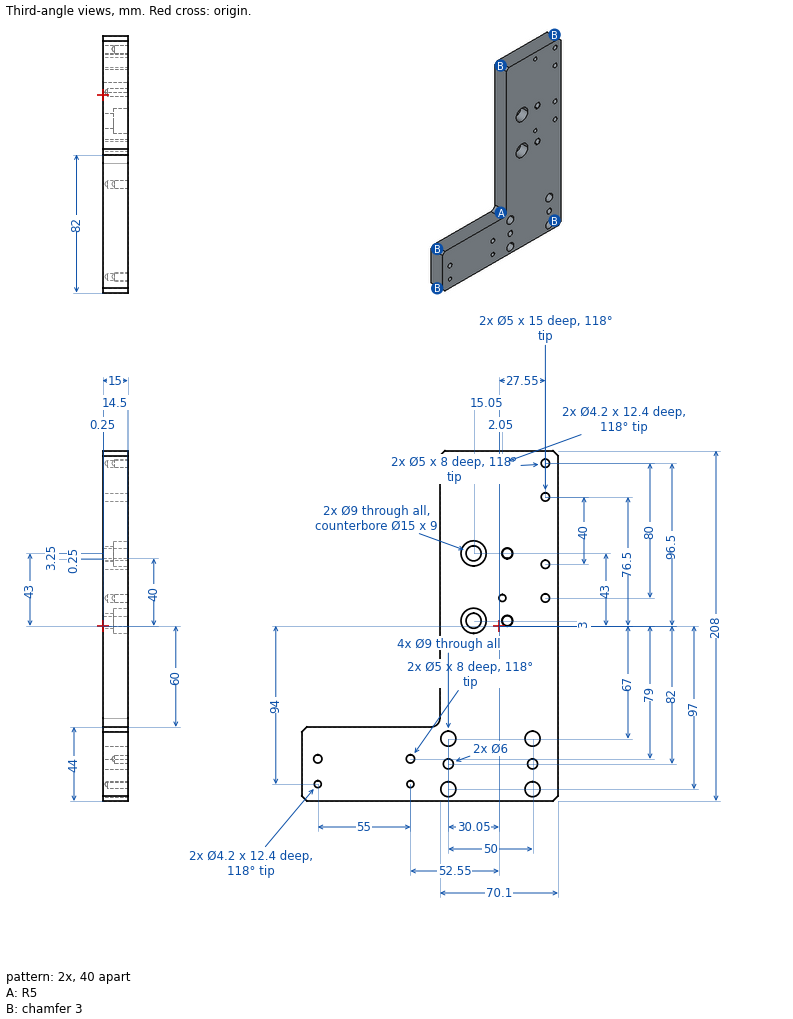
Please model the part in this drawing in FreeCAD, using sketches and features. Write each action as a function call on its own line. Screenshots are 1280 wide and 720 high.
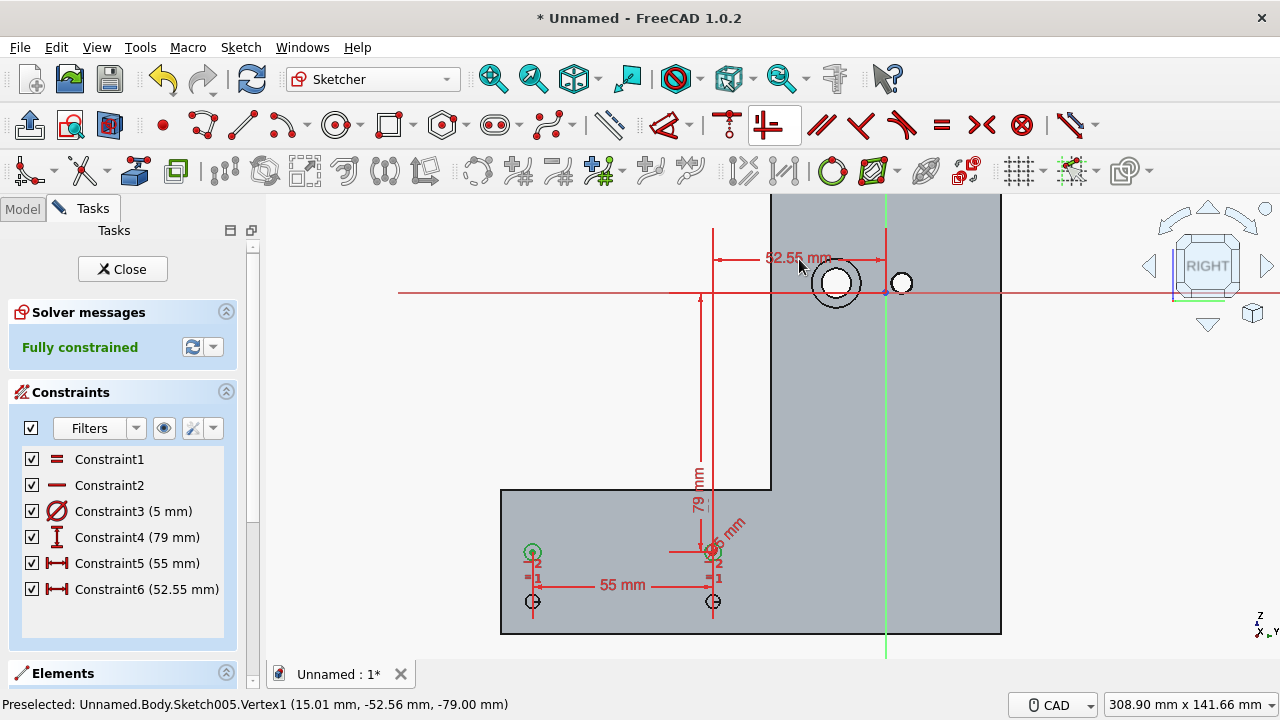
click(123, 269)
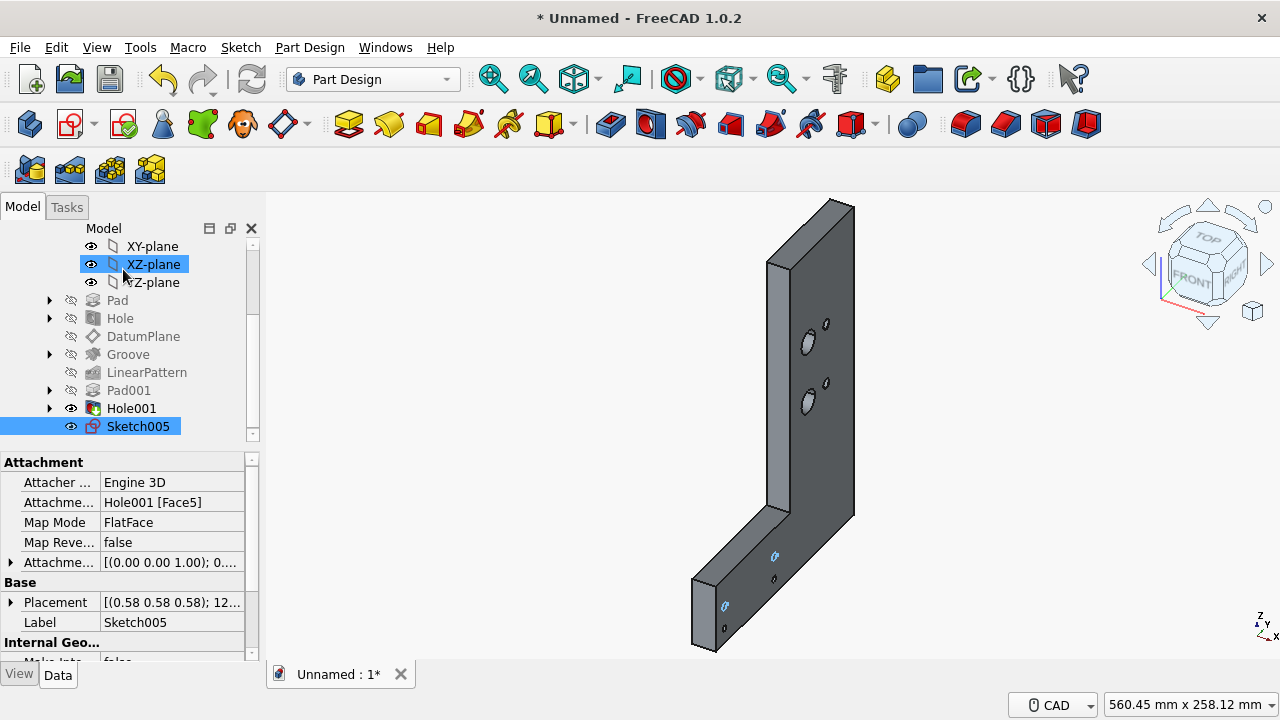
click(652, 124)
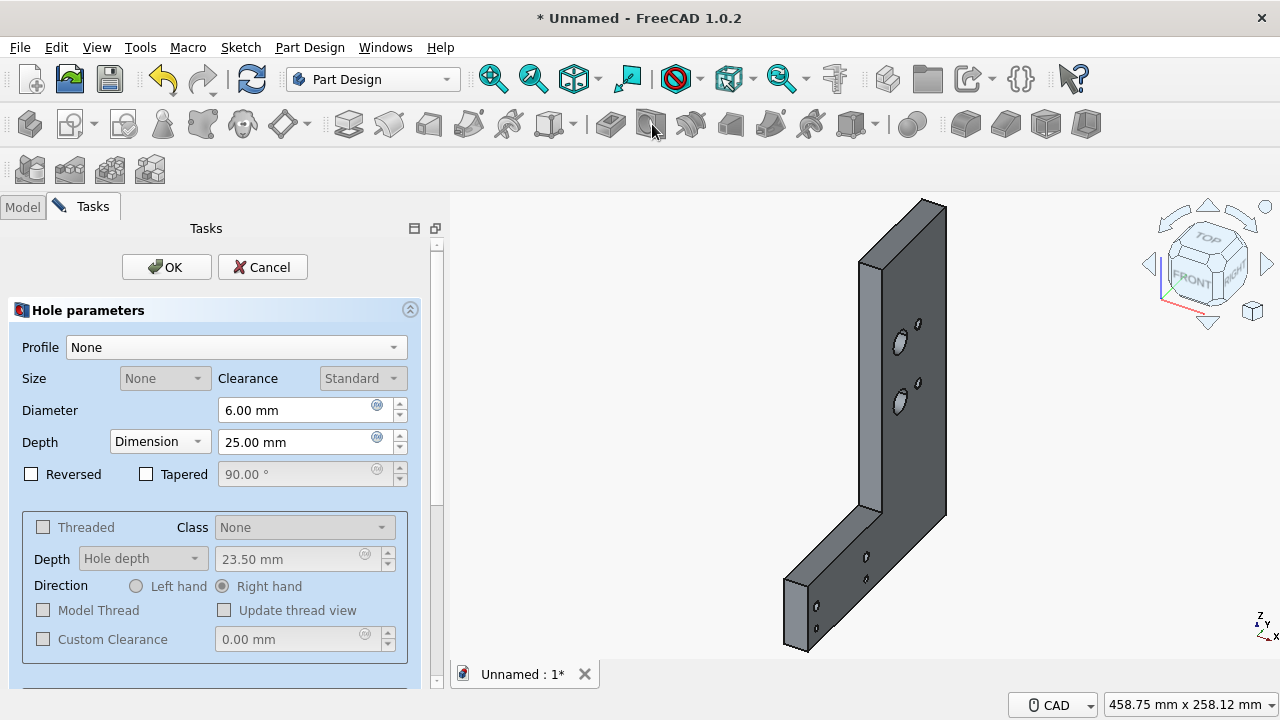
triple_click(305, 410)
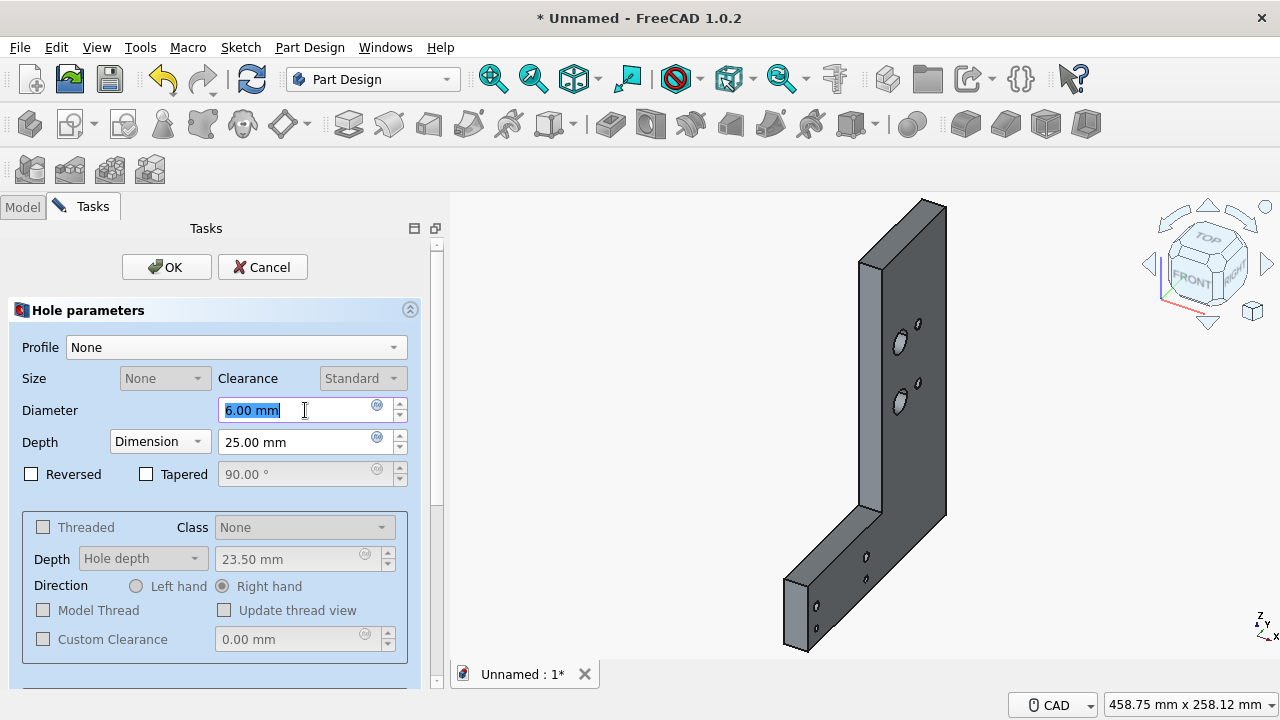
text(5)
key(Tab)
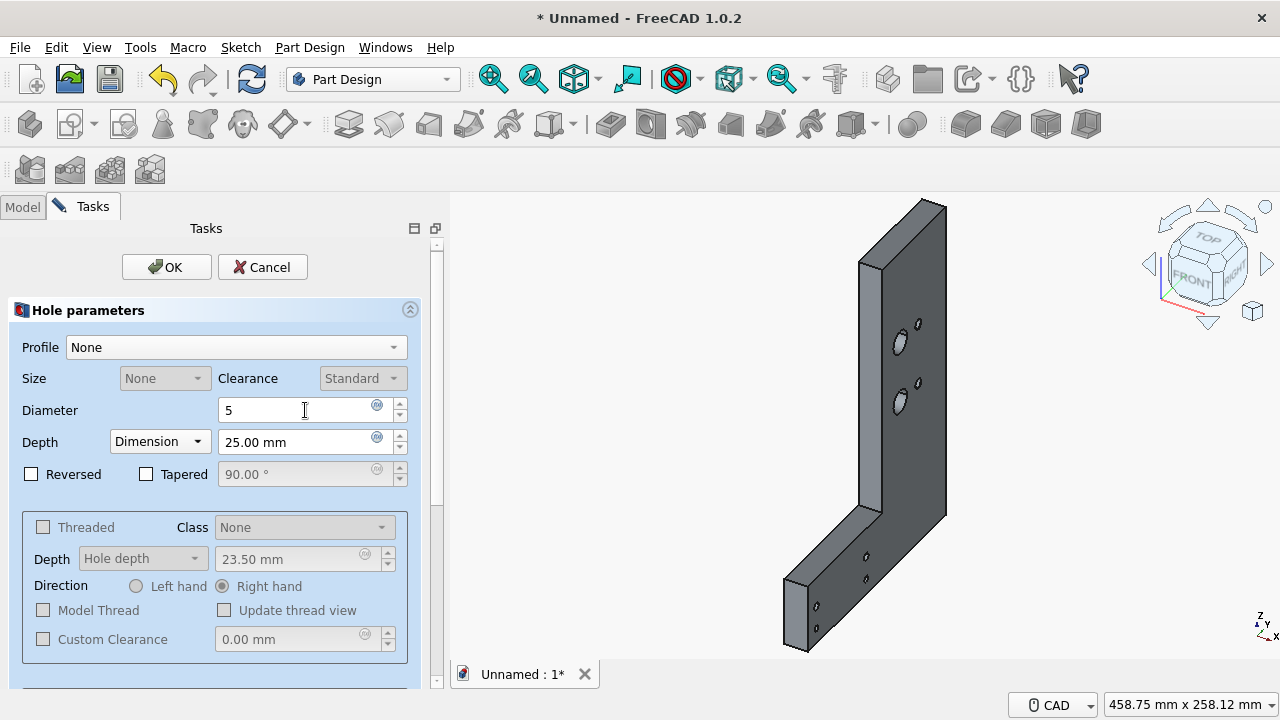
triple_click(305, 442)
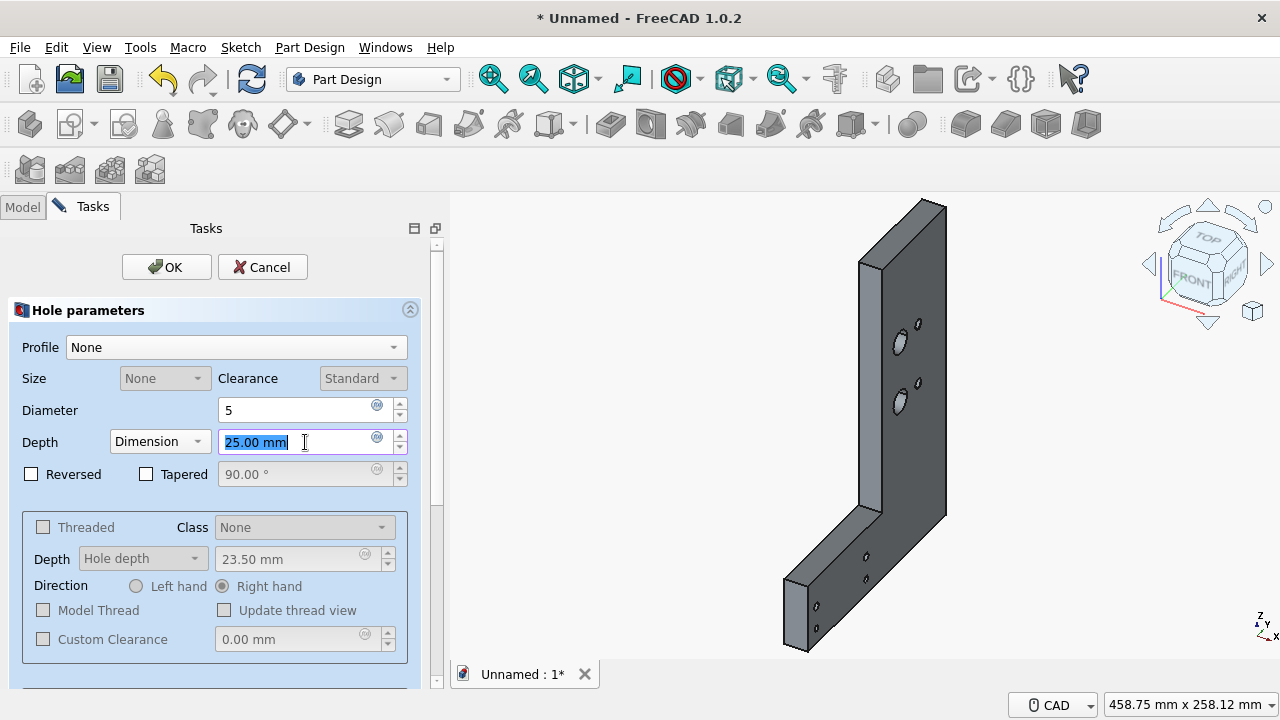
text(8)
key(Tab)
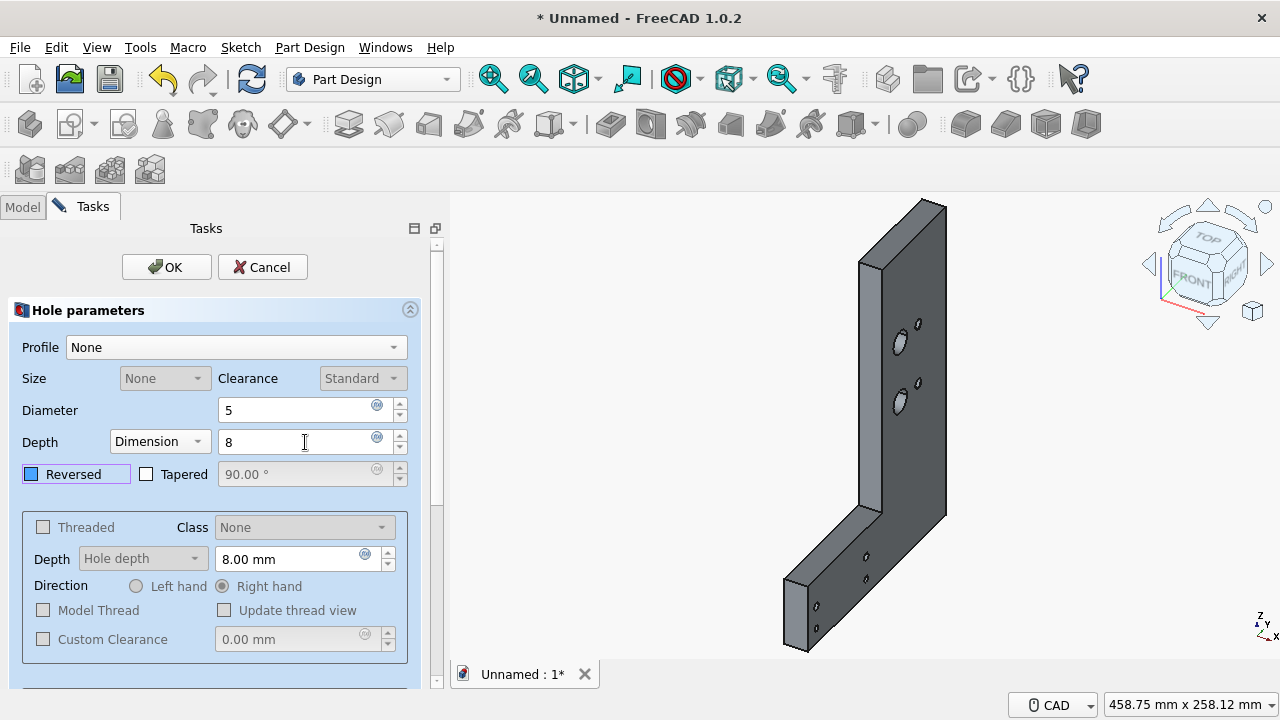
click(167, 267)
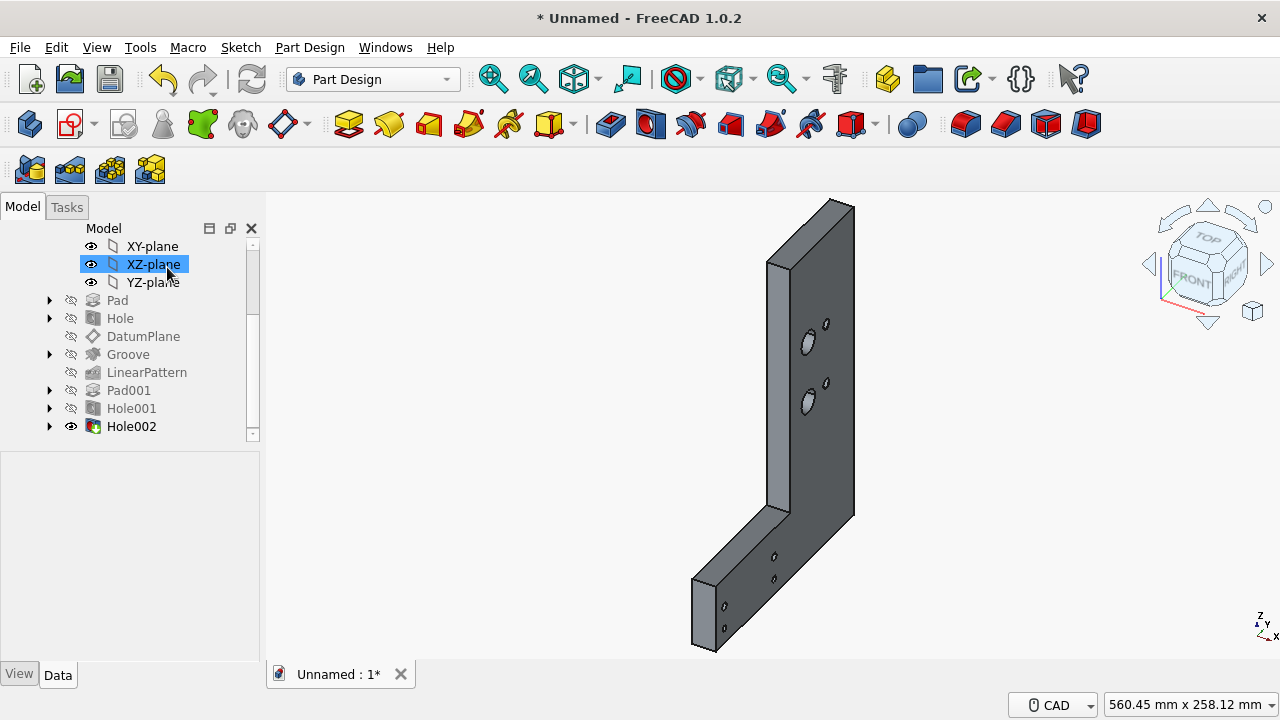
click(824, 477)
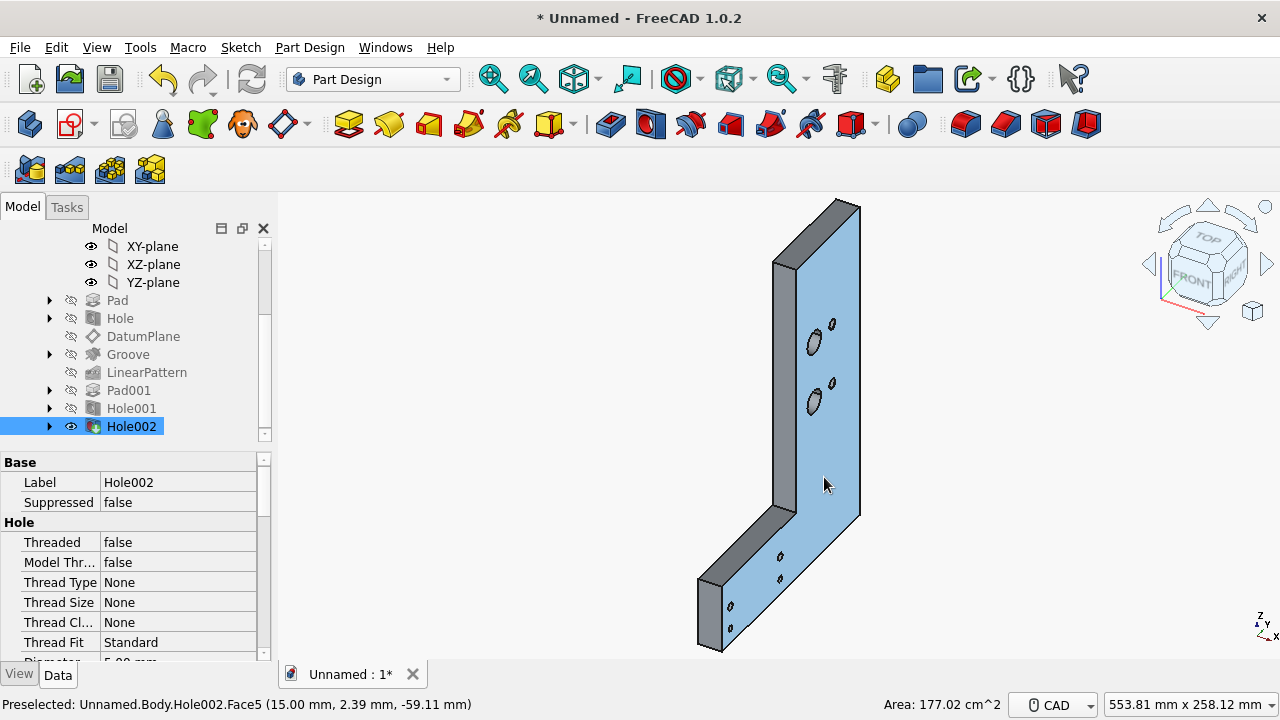
click(70, 124)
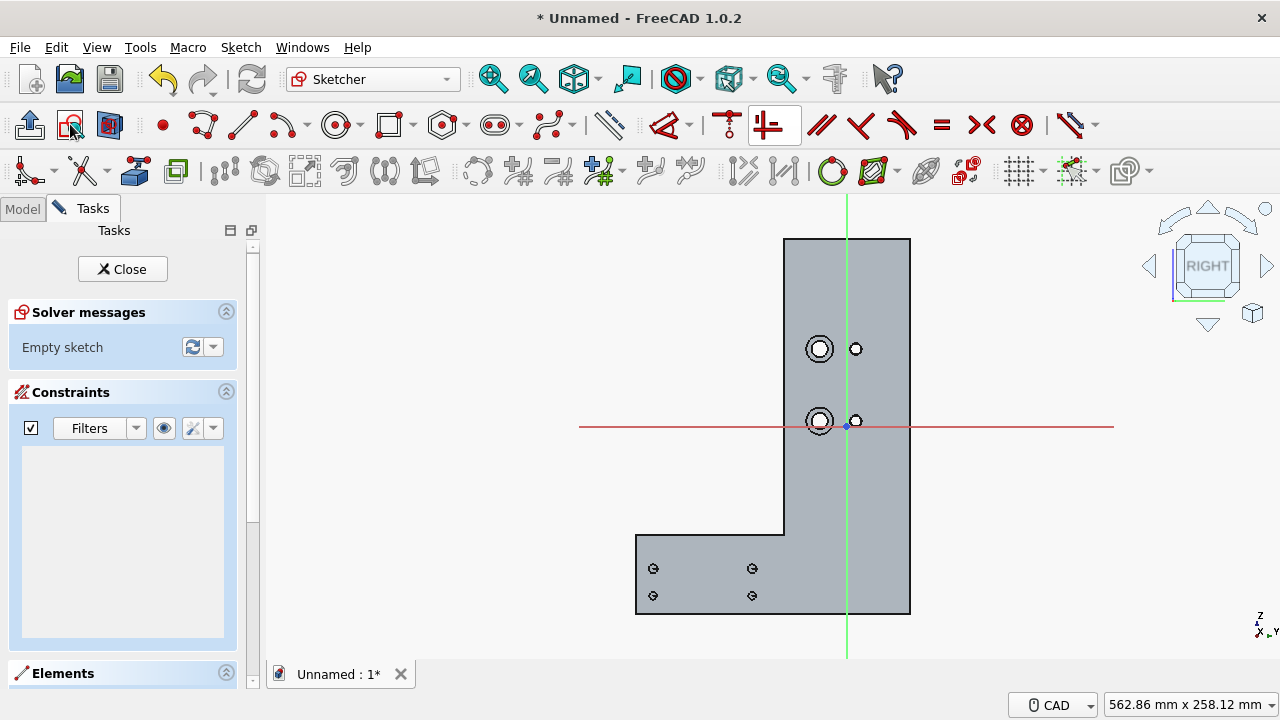
scroll(1012, 297, up, 4)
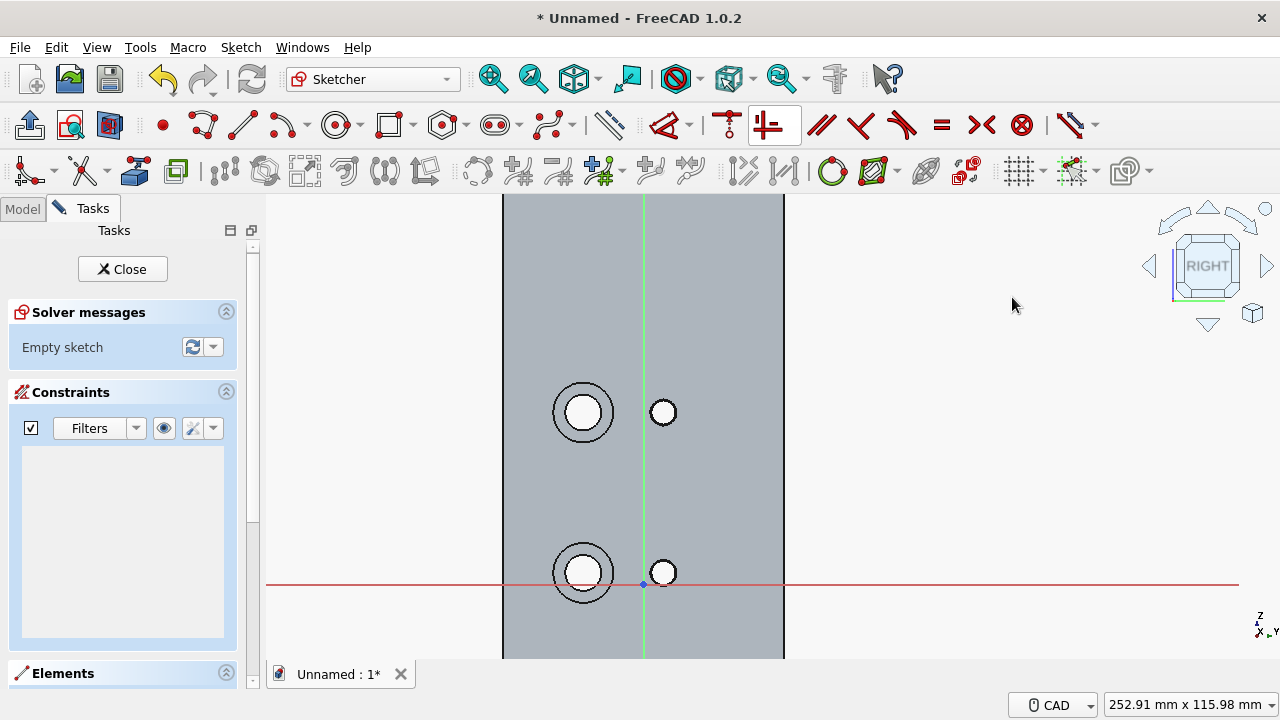
click(336, 126)